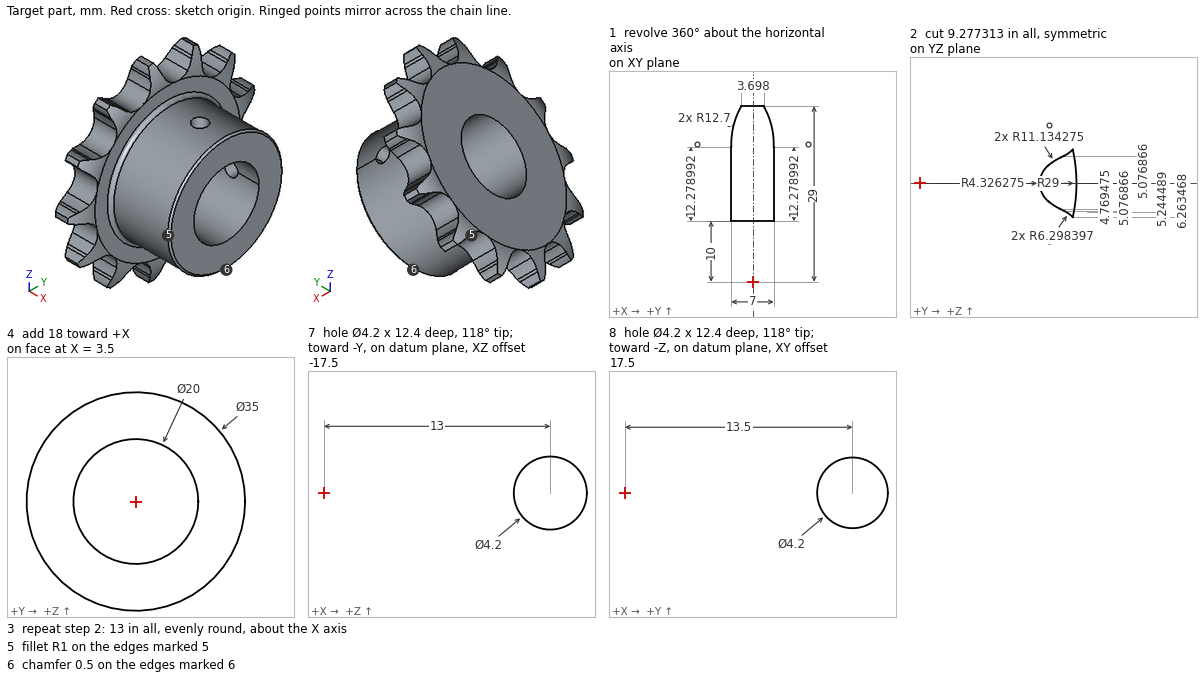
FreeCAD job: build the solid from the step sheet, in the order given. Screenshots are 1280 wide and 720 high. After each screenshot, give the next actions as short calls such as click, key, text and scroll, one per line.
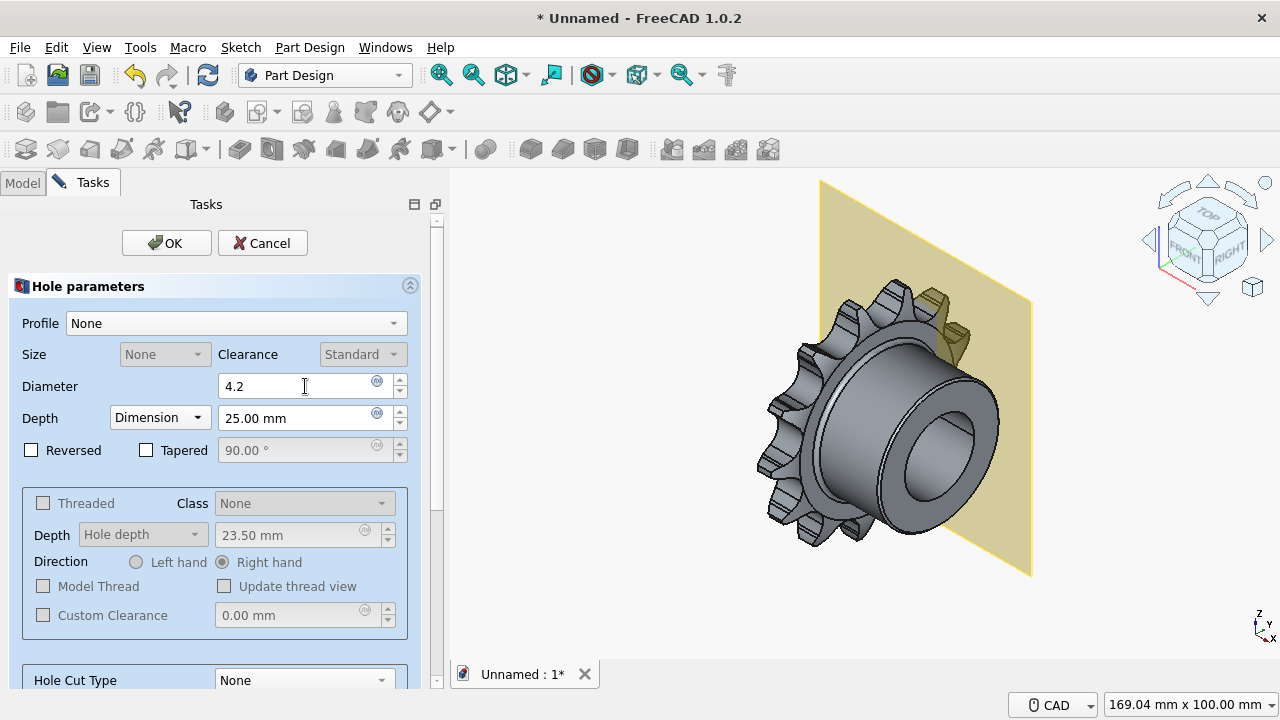
triple_click(305, 418)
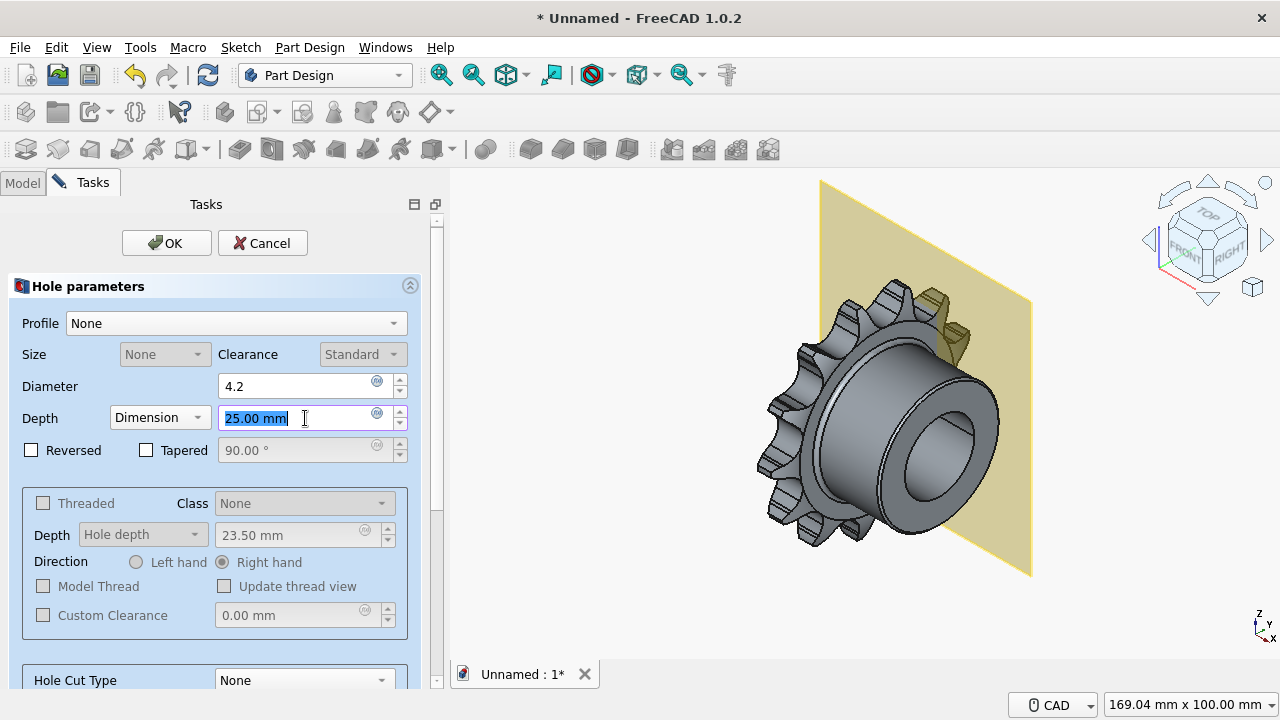
text(12.4)
key(Tab)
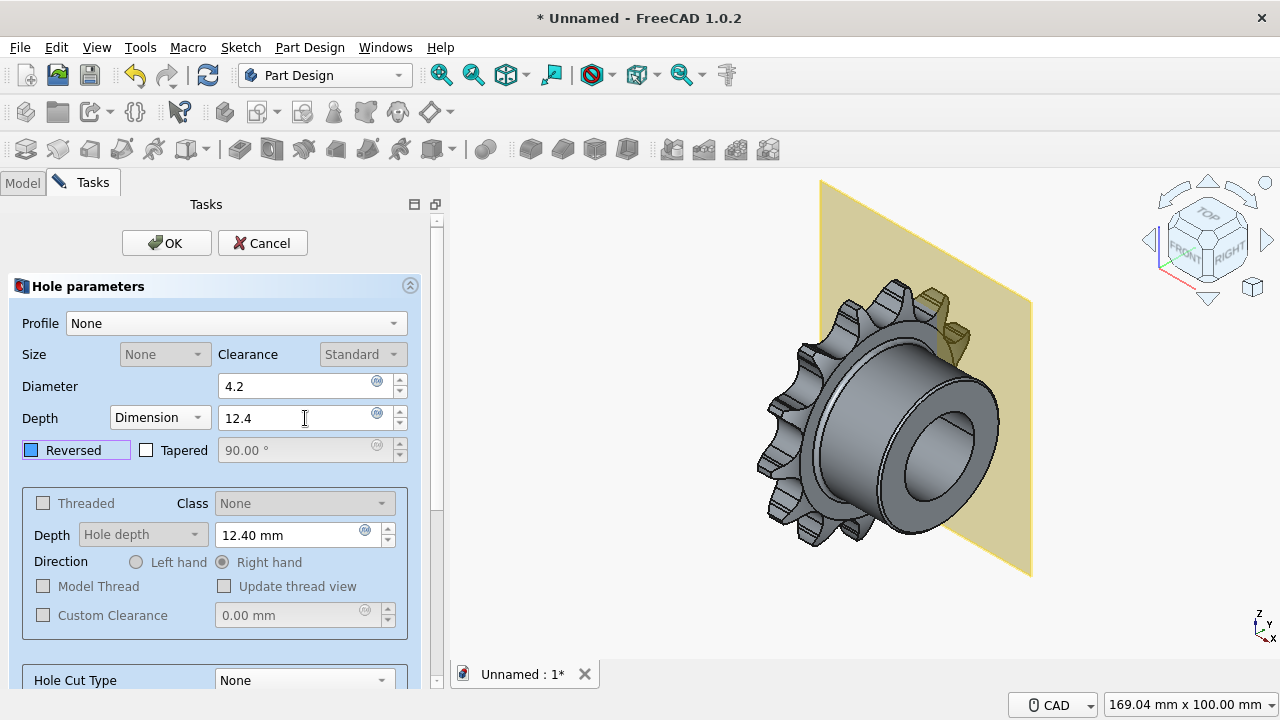
click(30, 450)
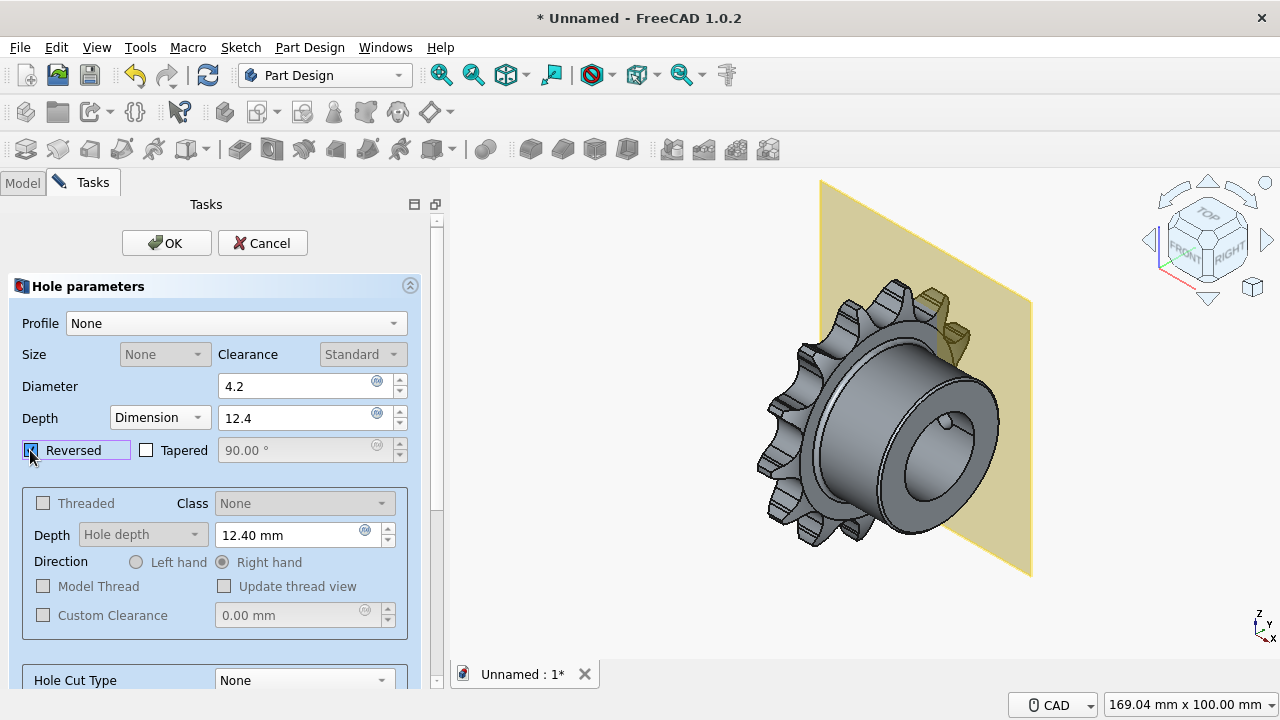
click(167, 243)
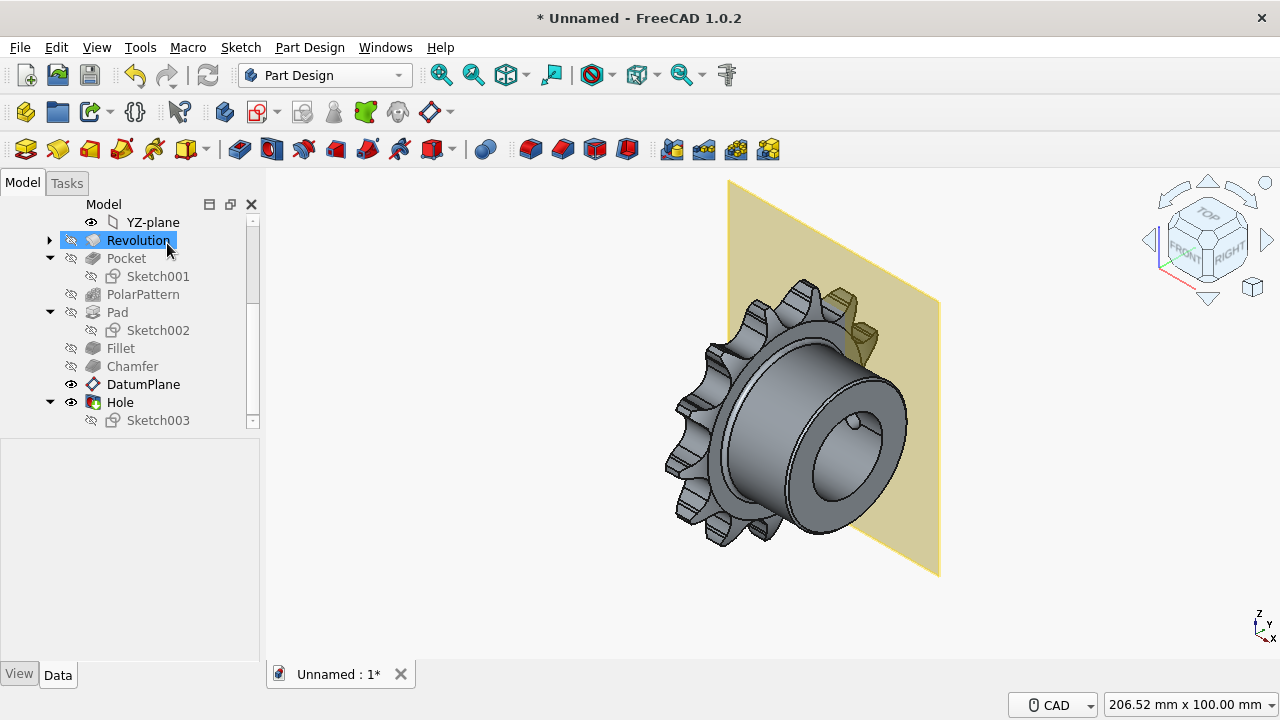
click(116, 384)
key(space)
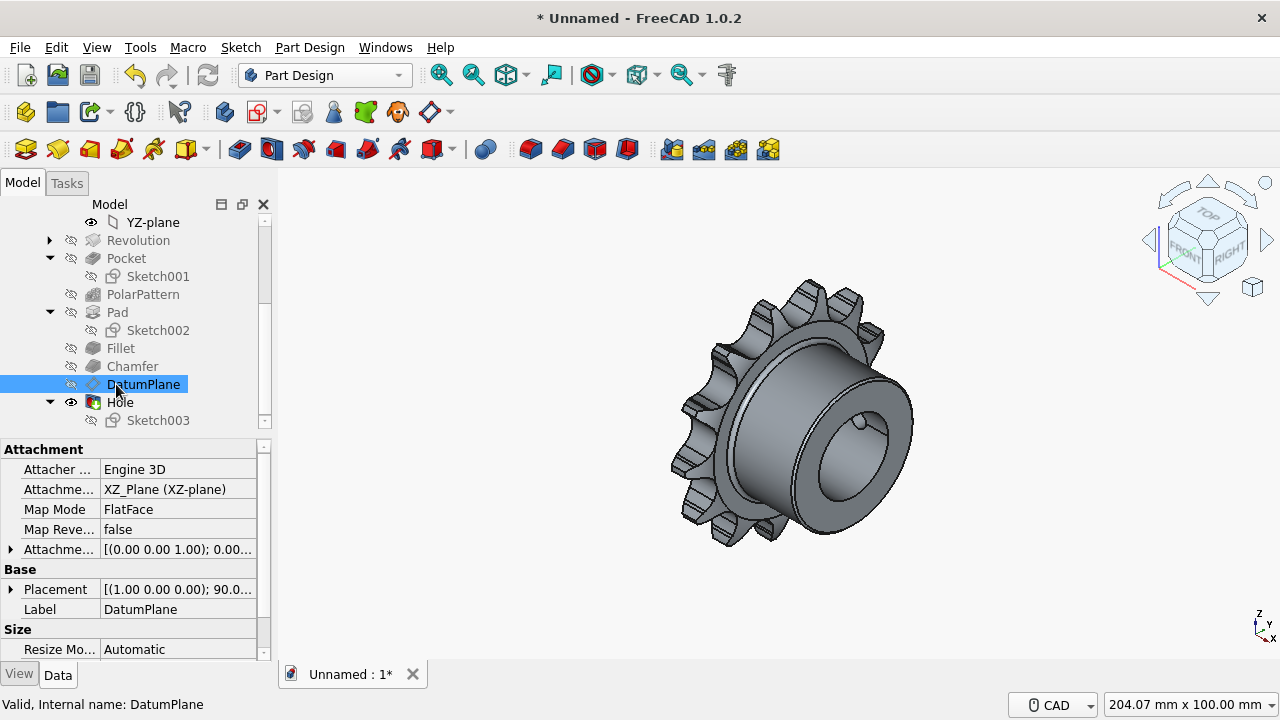
scroll(160, 326, down, 3)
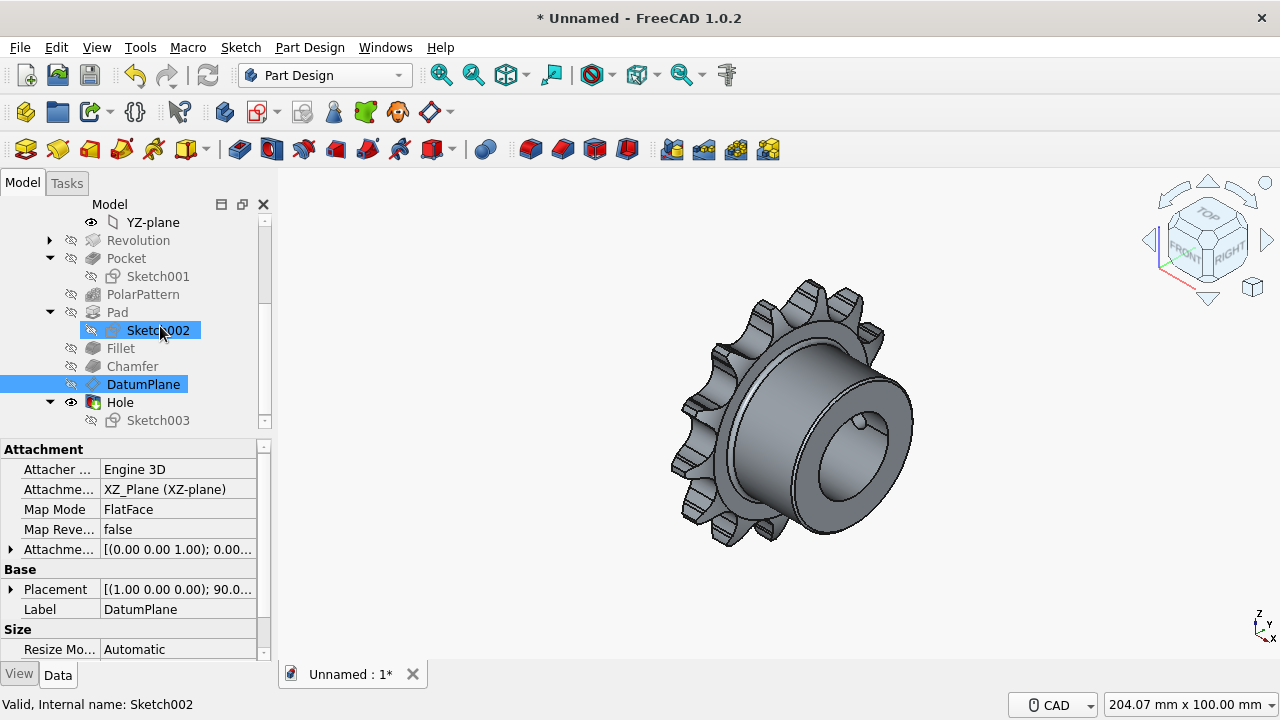
scroll(160, 326, up, 15)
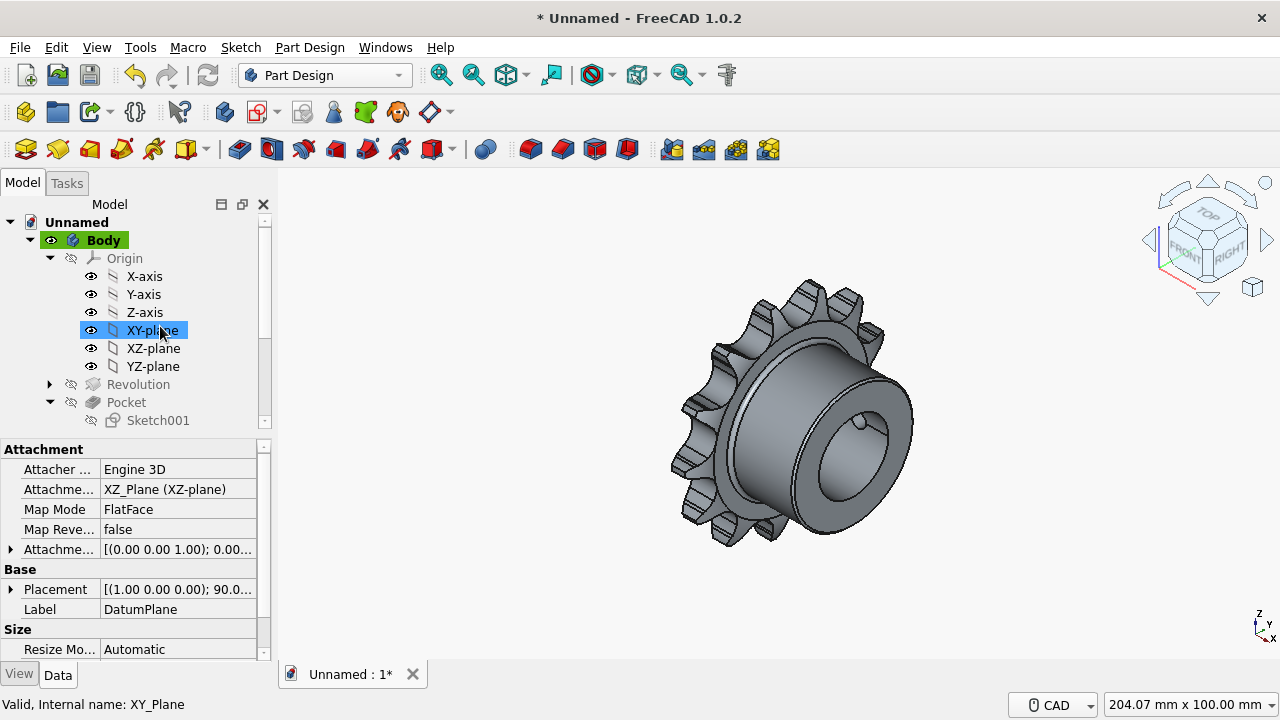
click(136, 330)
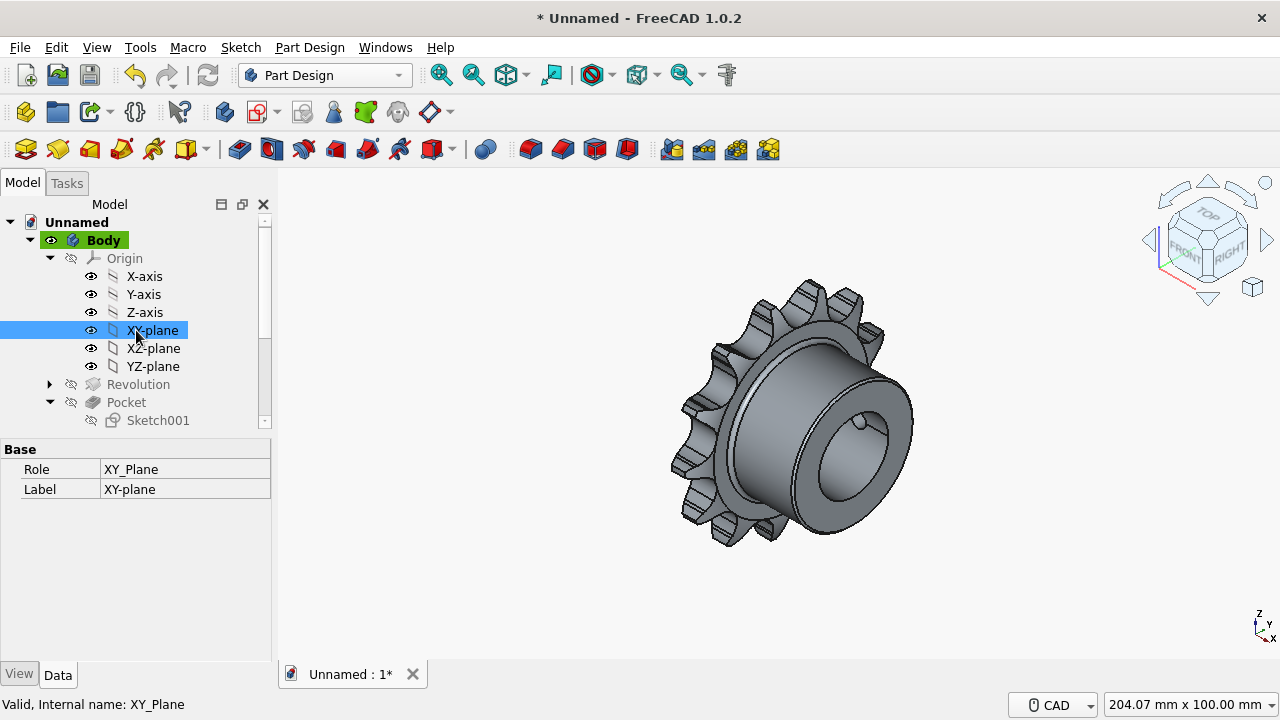
click(430, 112)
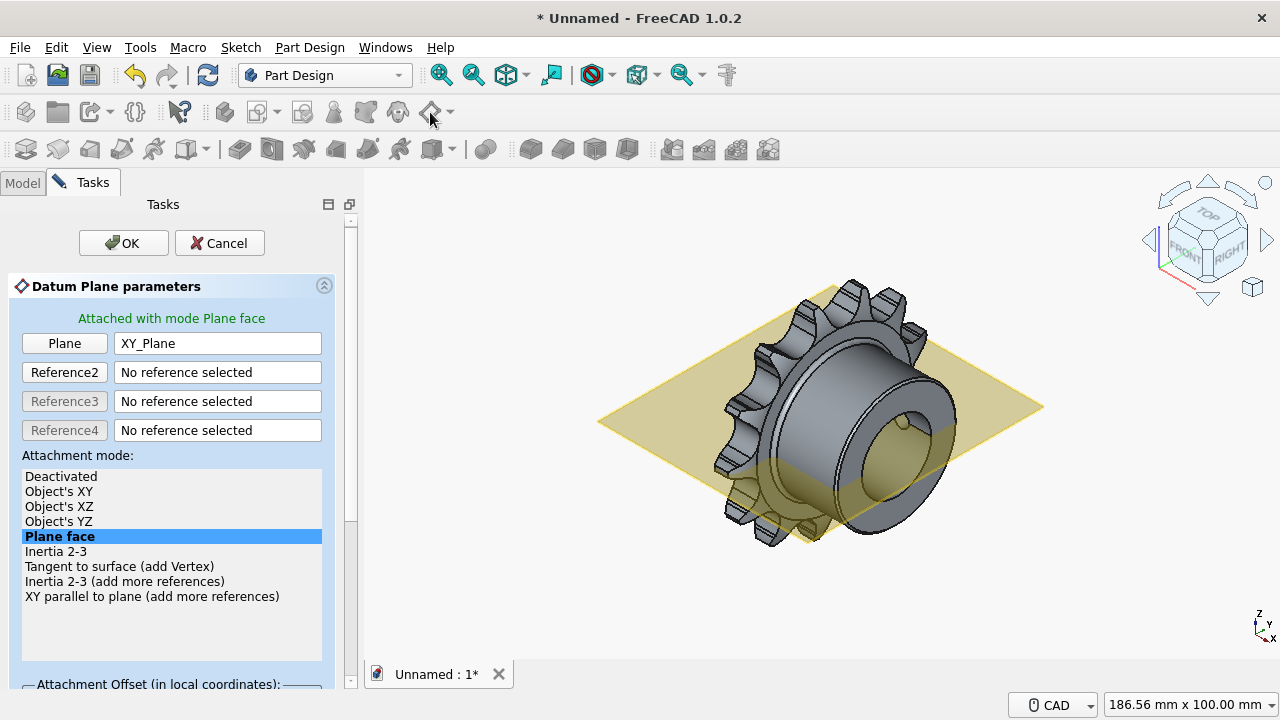
scroll(351, 451, down, 3)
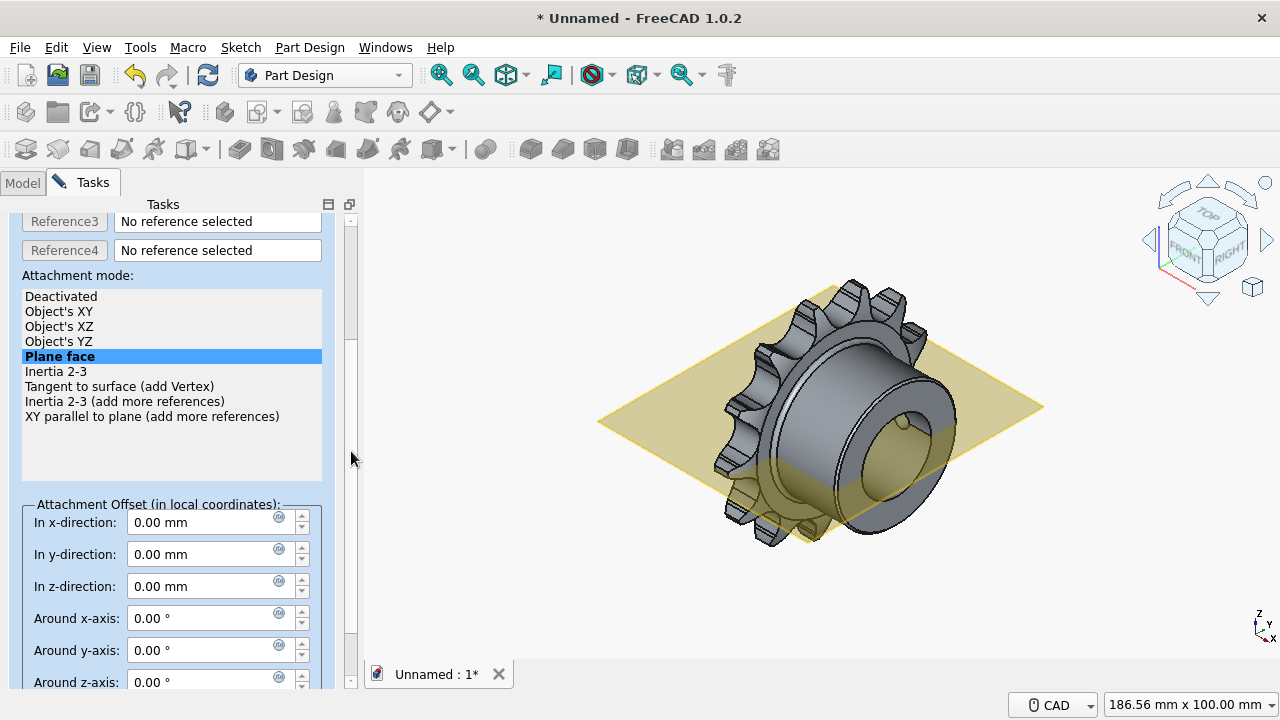
triple_click(210, 586)